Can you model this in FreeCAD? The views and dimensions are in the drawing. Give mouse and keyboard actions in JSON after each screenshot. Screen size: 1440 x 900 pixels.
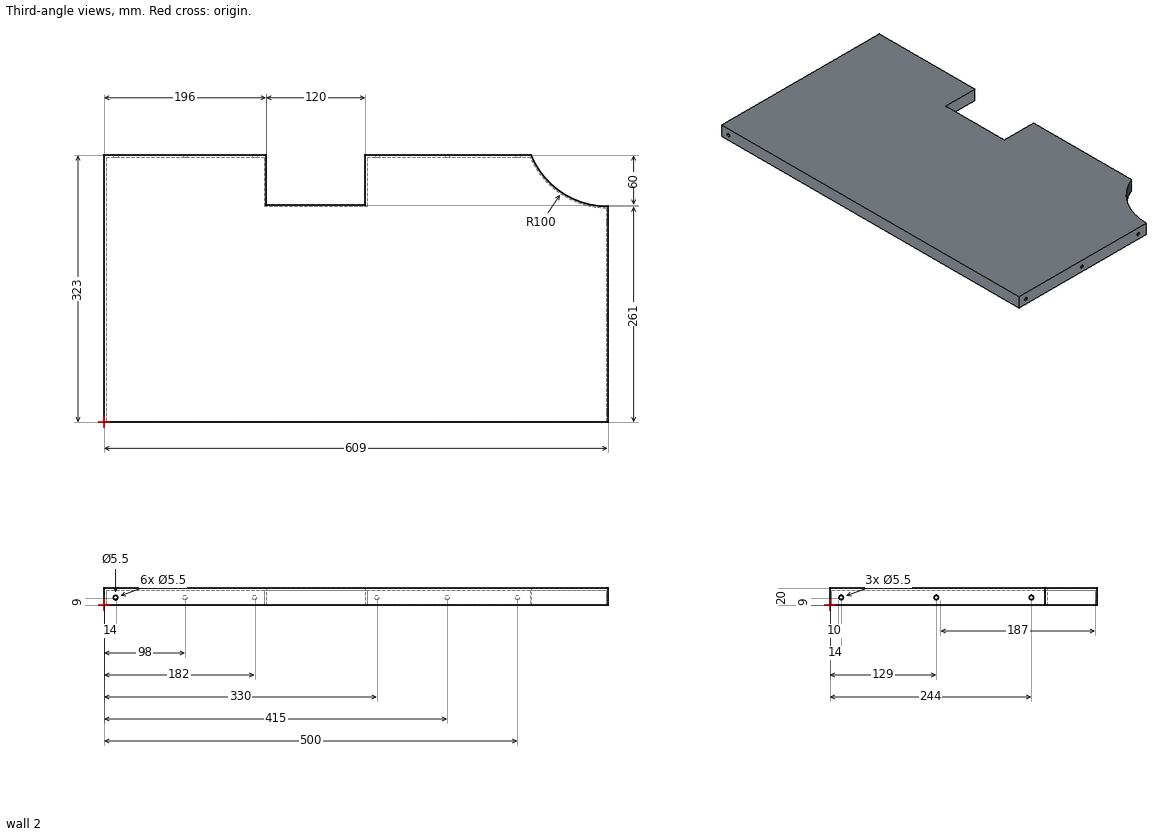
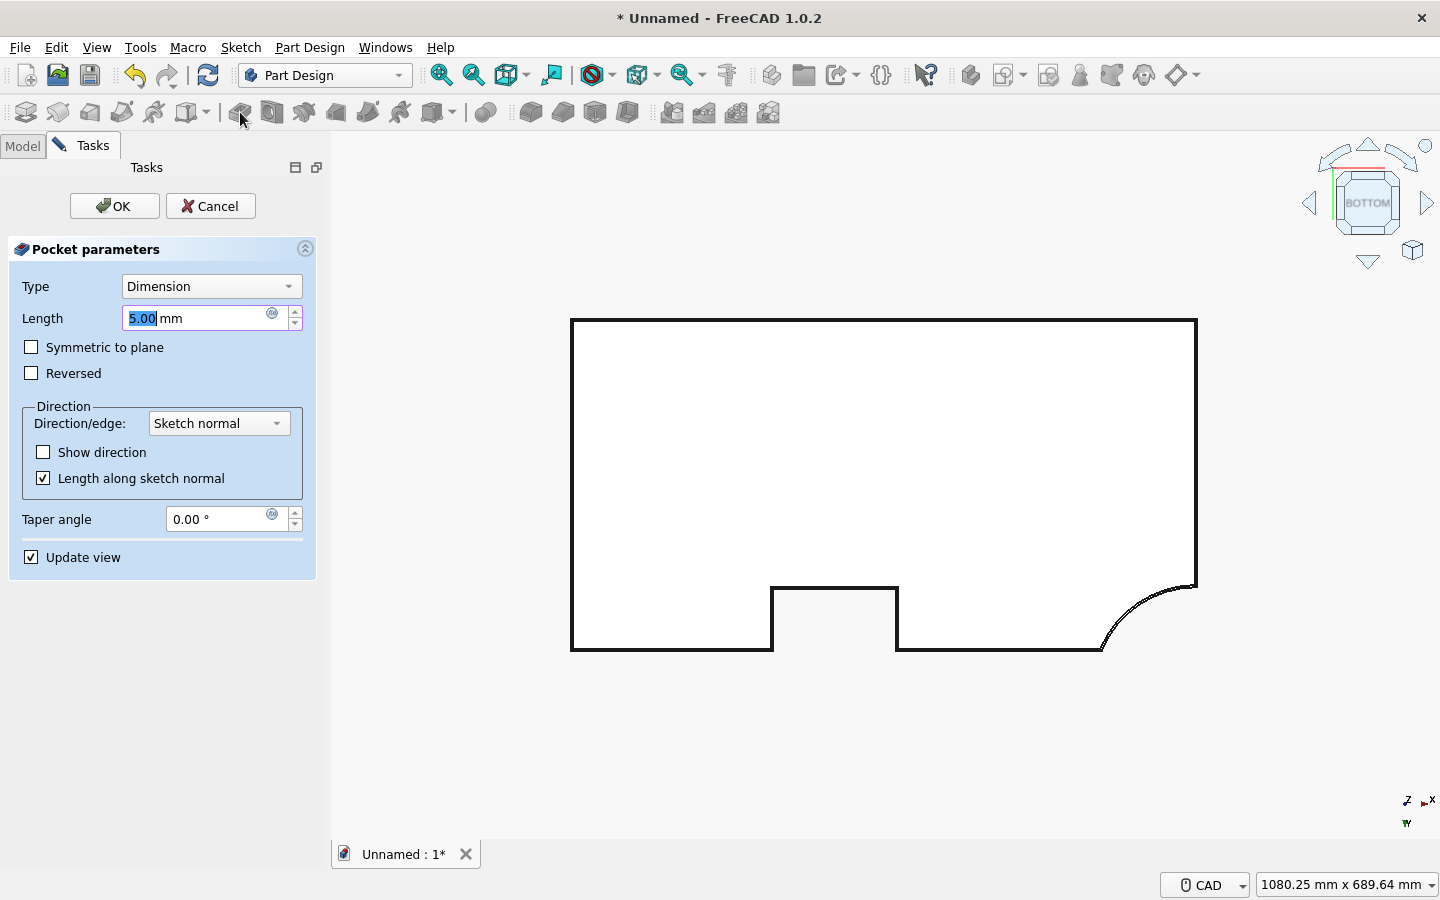
{"action": "type", "text": "10"}
{"action": "key", "text": "Tab"}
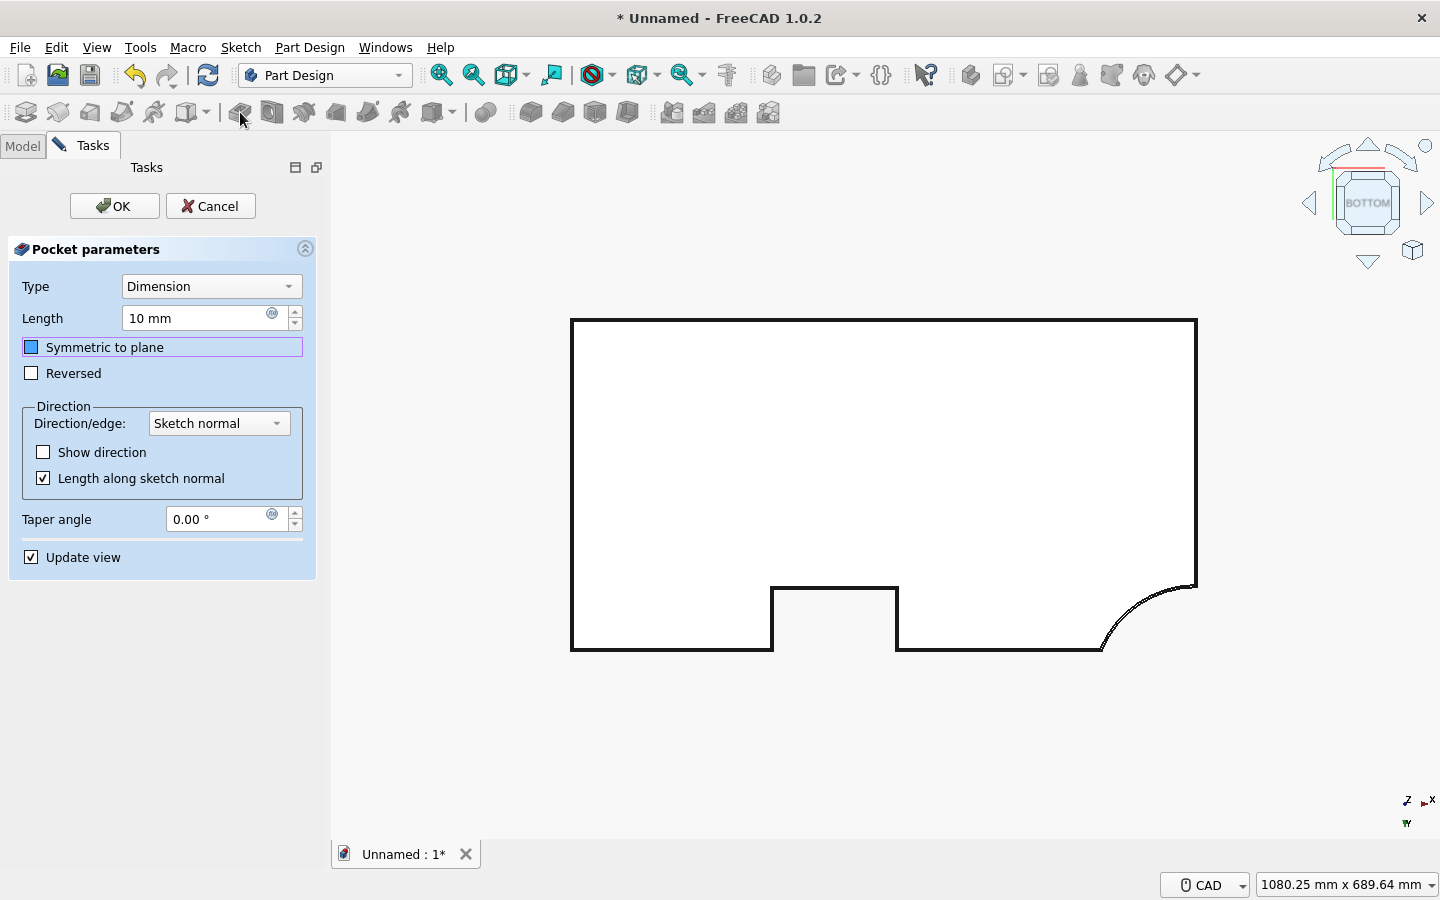
{"action": "left_click", "coordinate": [115, 206]}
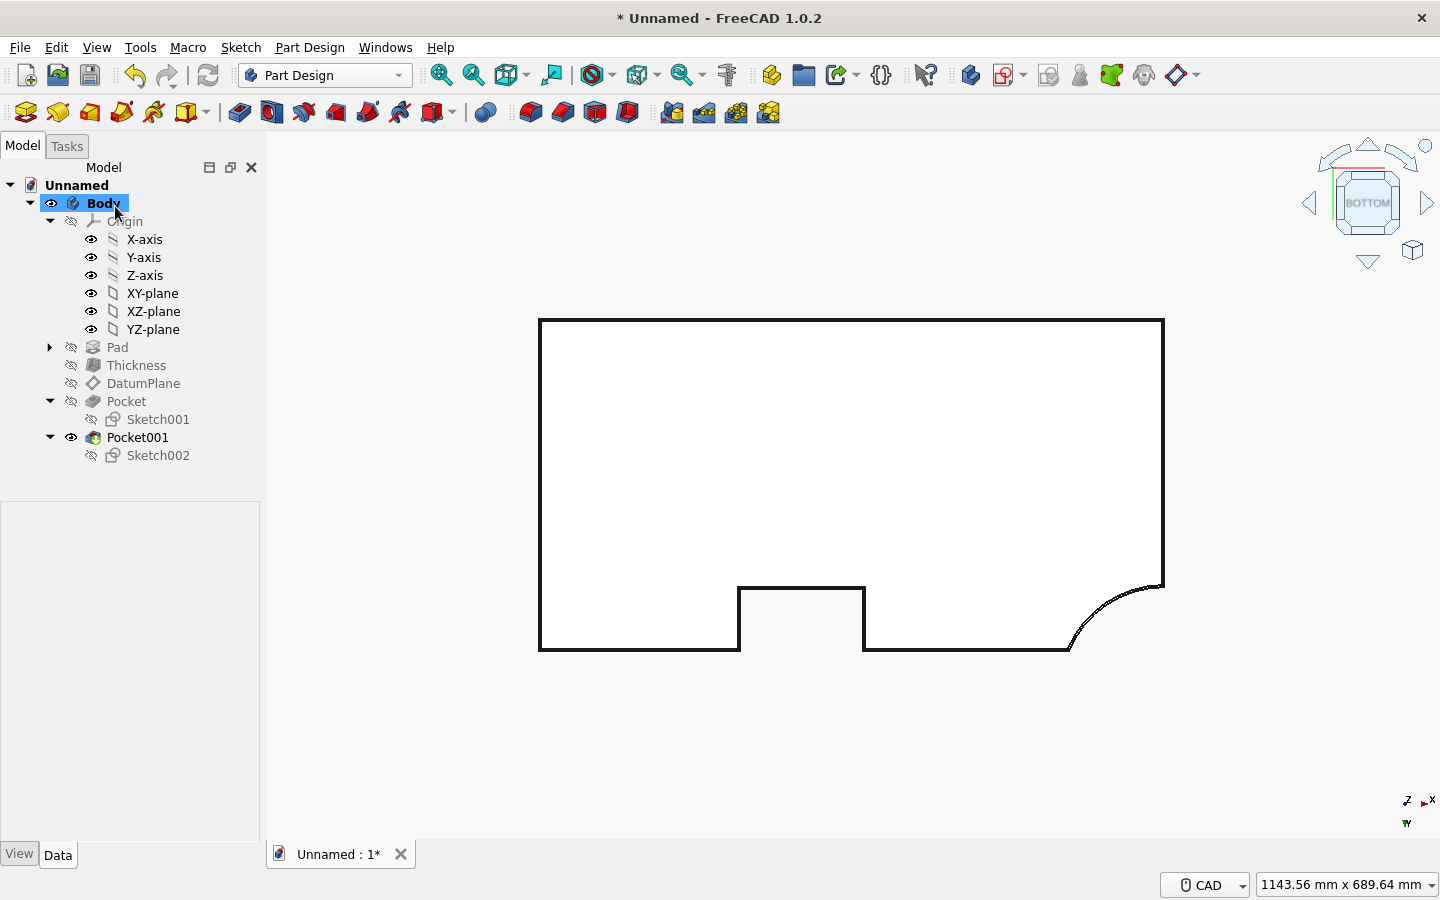
{"action": "left_click", "coordinate": [136, 329]}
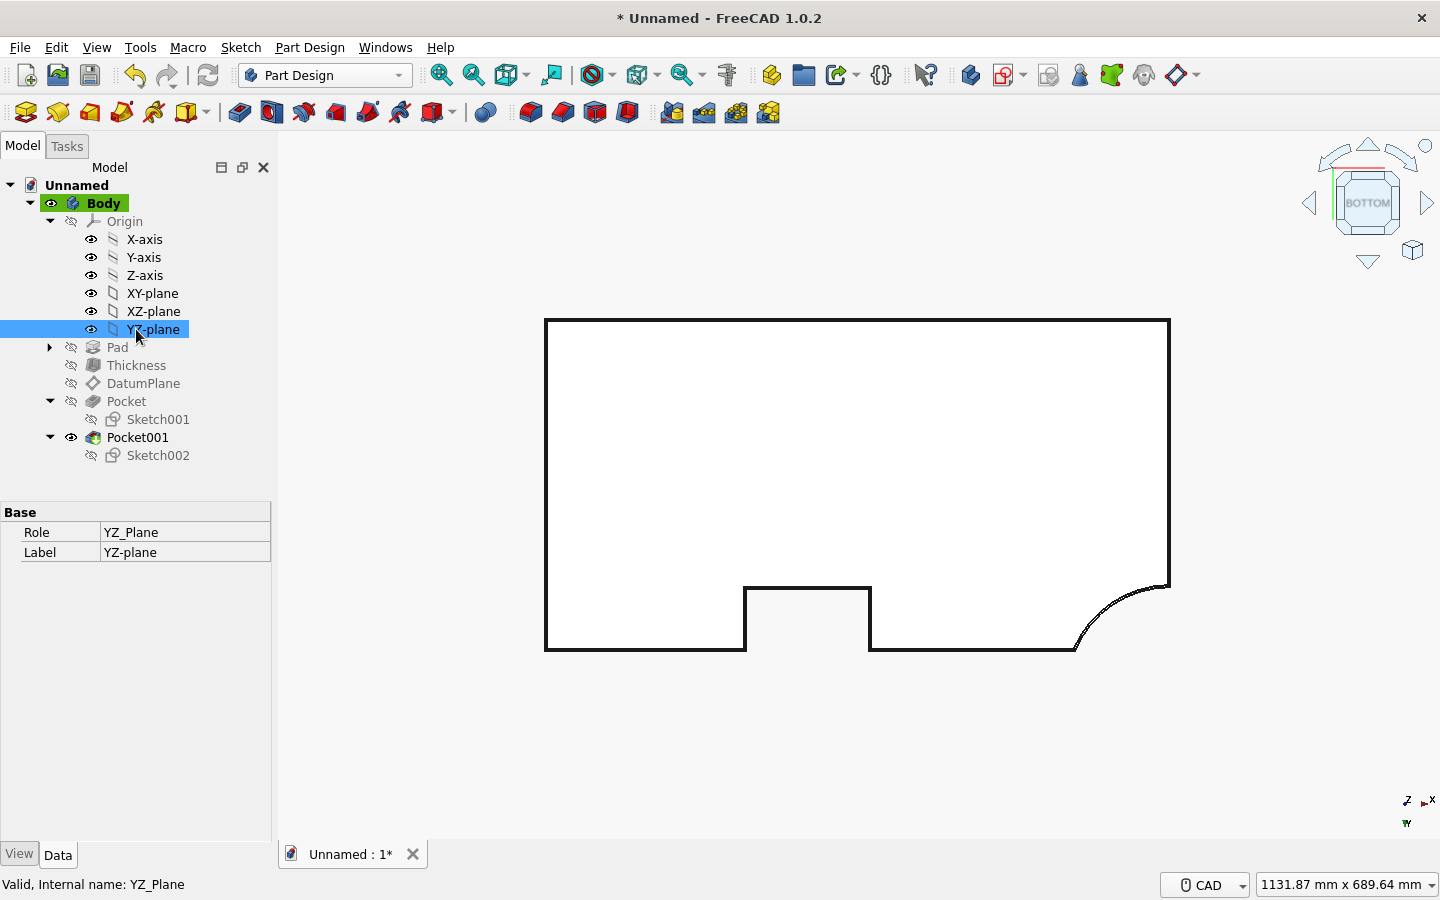
{"action": "left_click", "coordinate": [1176, 76]}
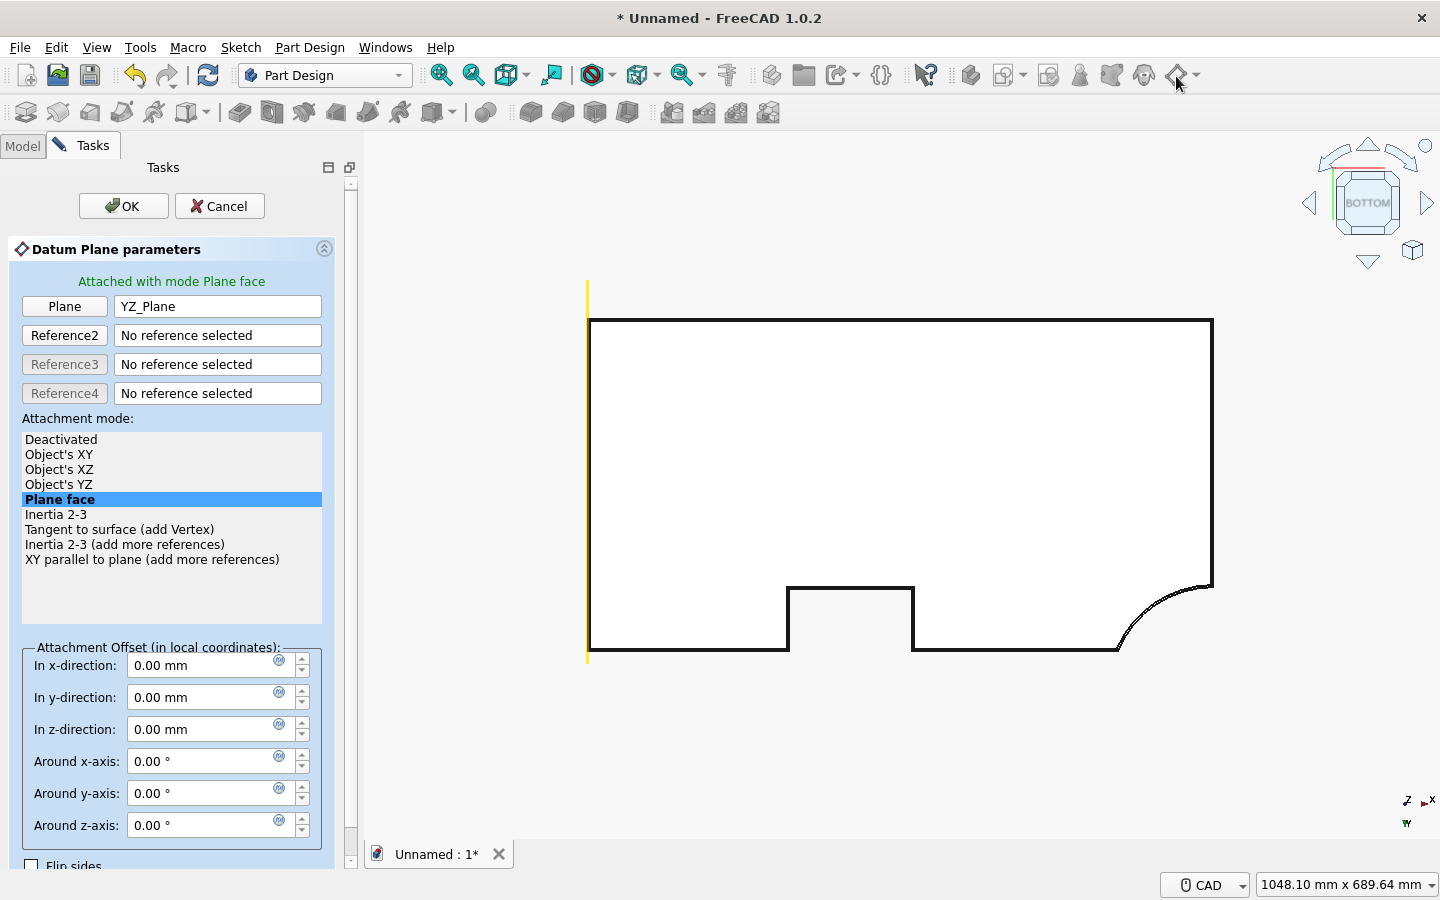
{"action": "triple_click", "coordinate": [210, 729]}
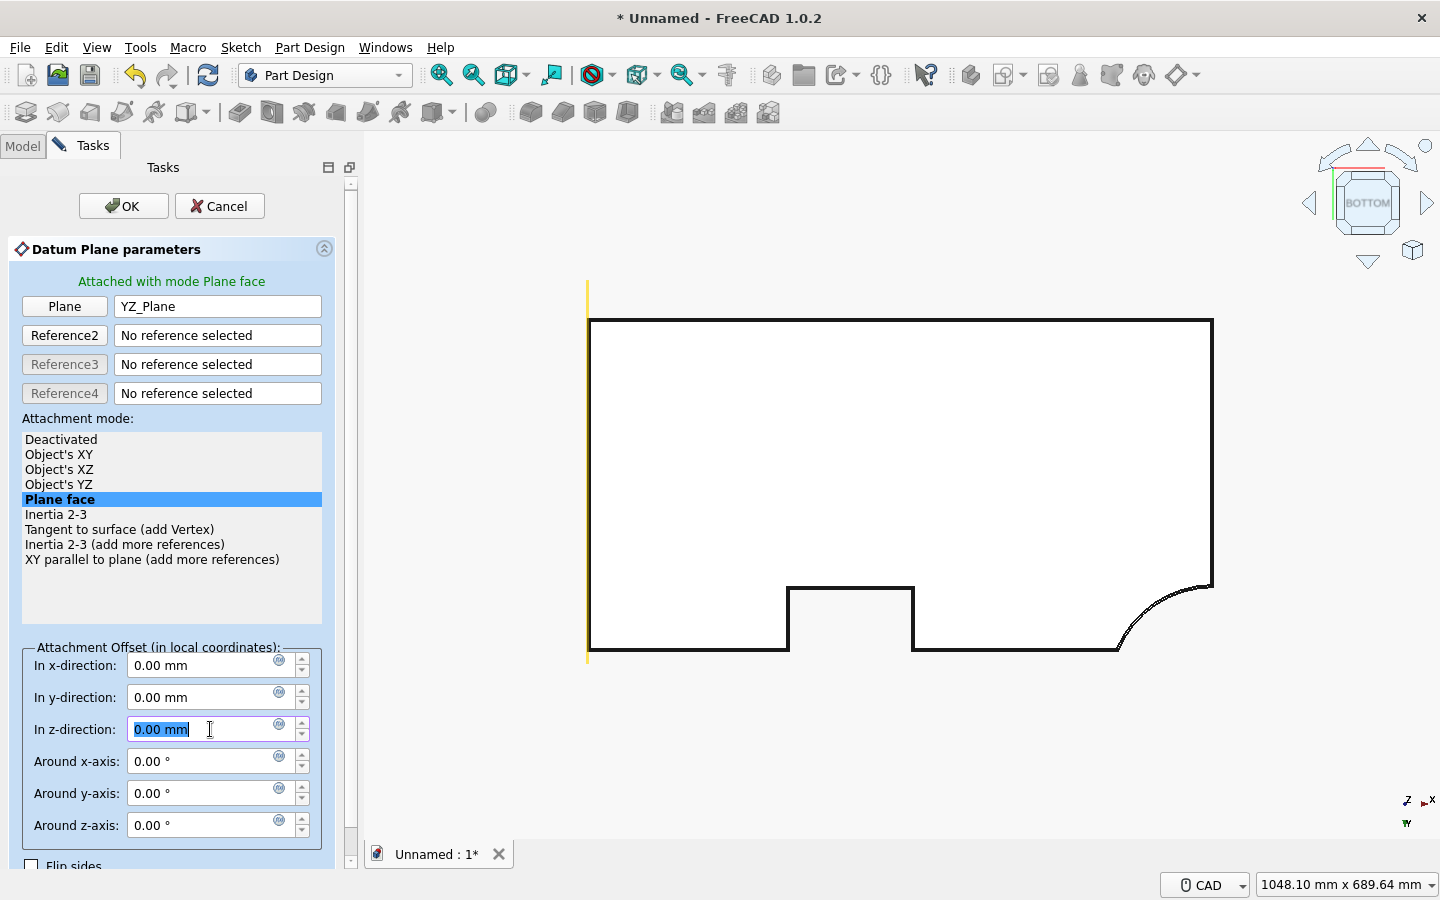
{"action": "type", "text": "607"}
{"action": "key", "text": "Tab"}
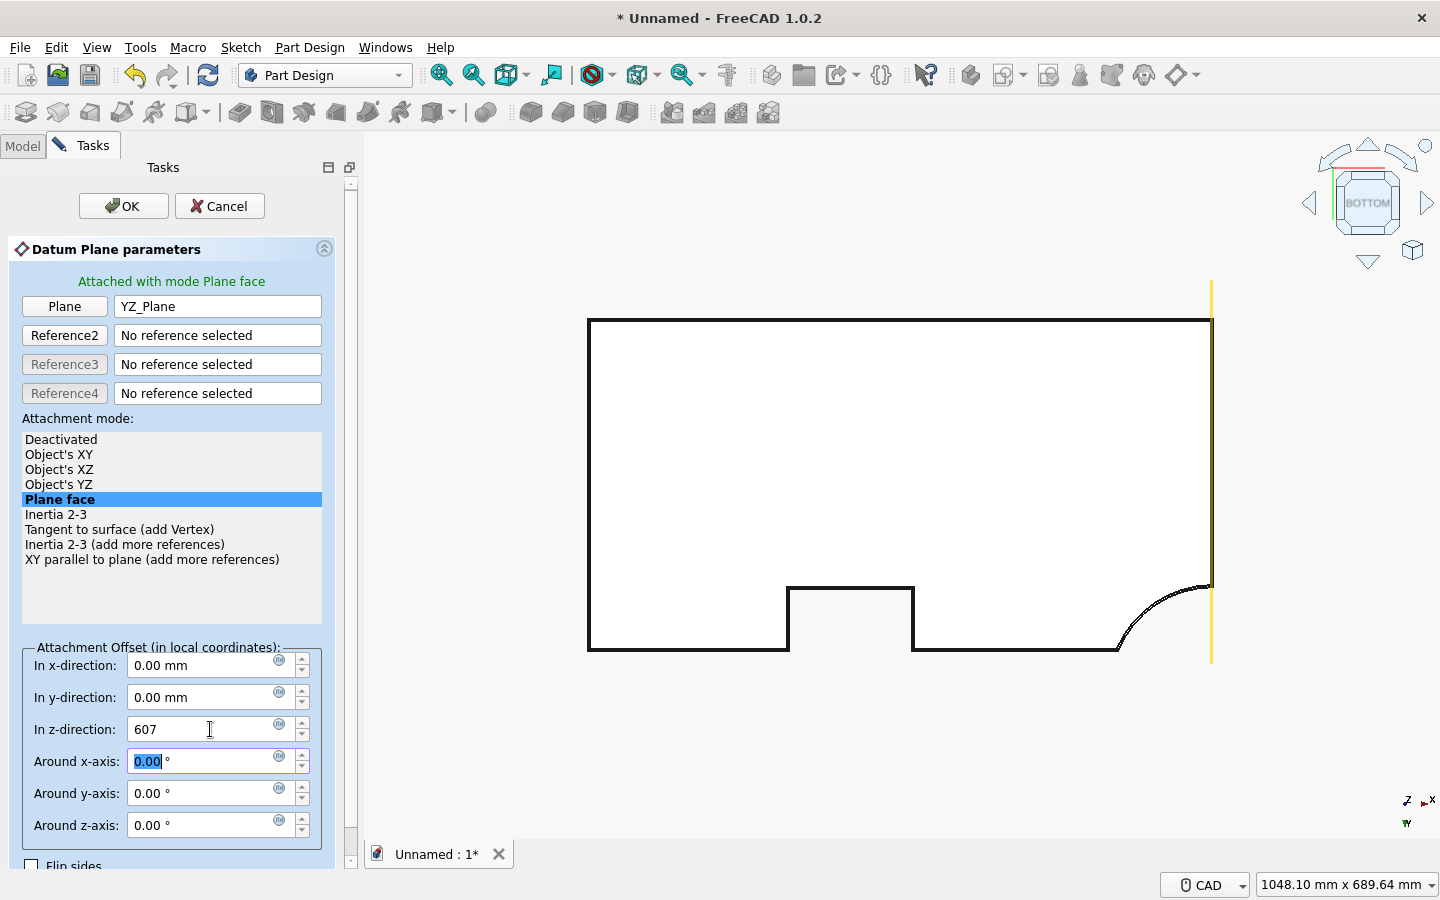
{"action": "left_click", "coordinate": [124, 206]}